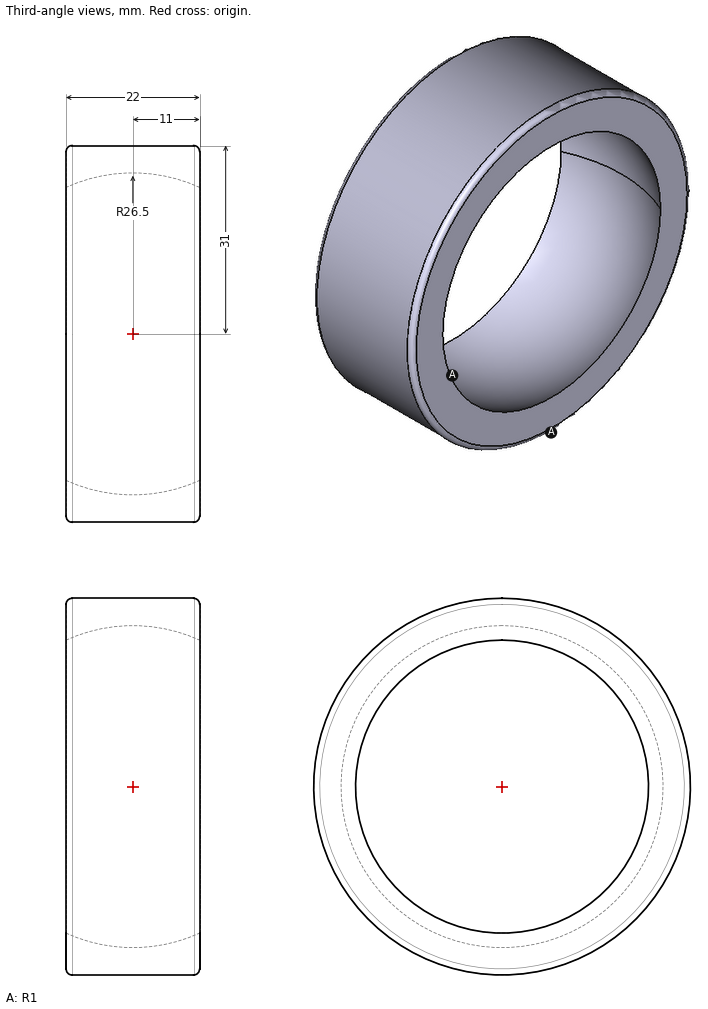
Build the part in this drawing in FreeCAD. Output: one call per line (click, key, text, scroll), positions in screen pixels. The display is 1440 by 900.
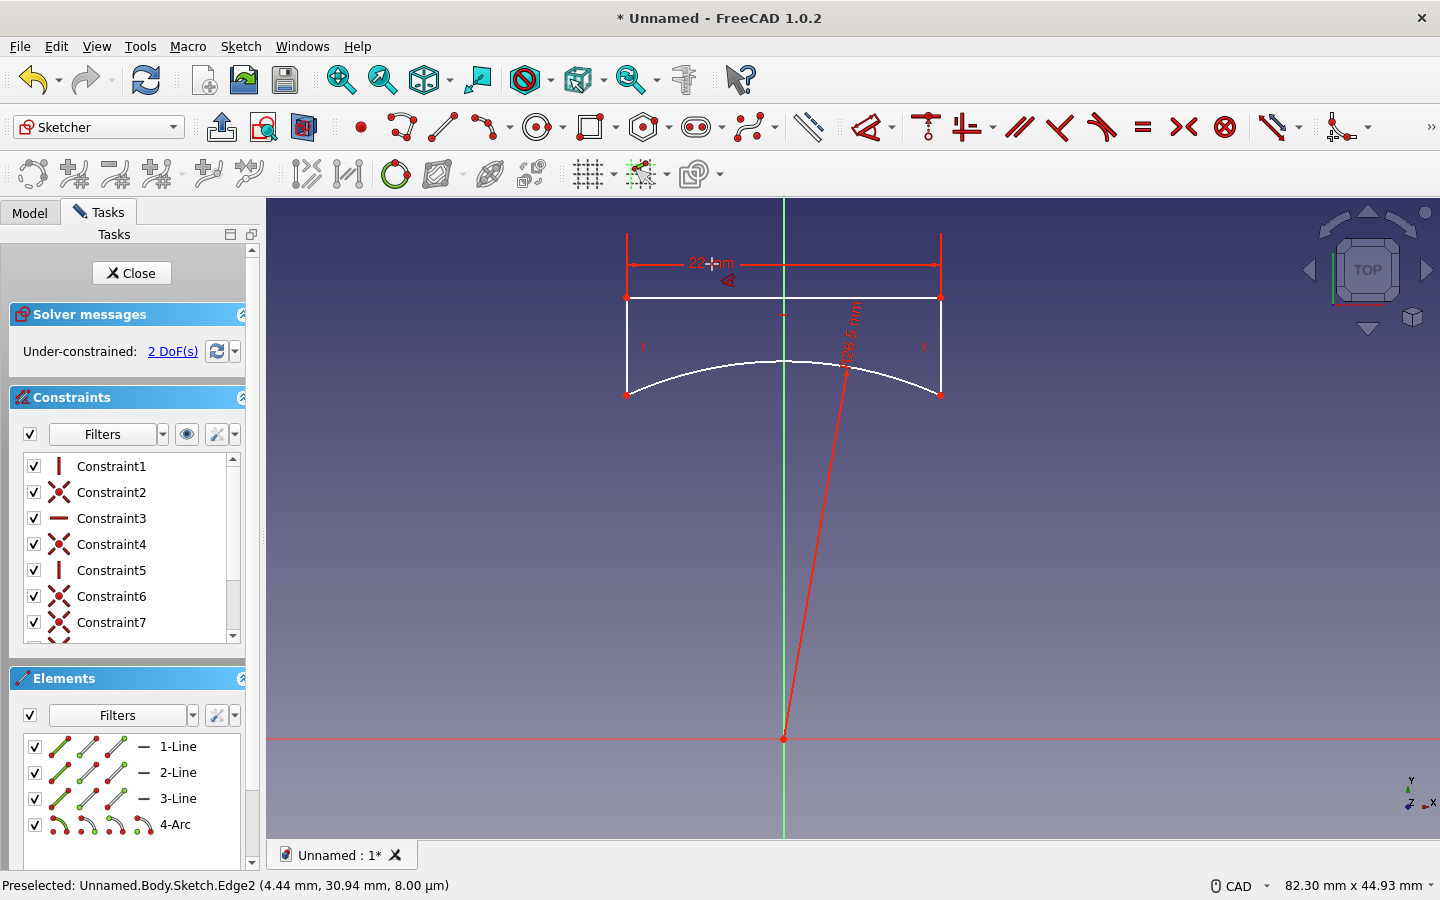
click(941, 396)
click(862, 773)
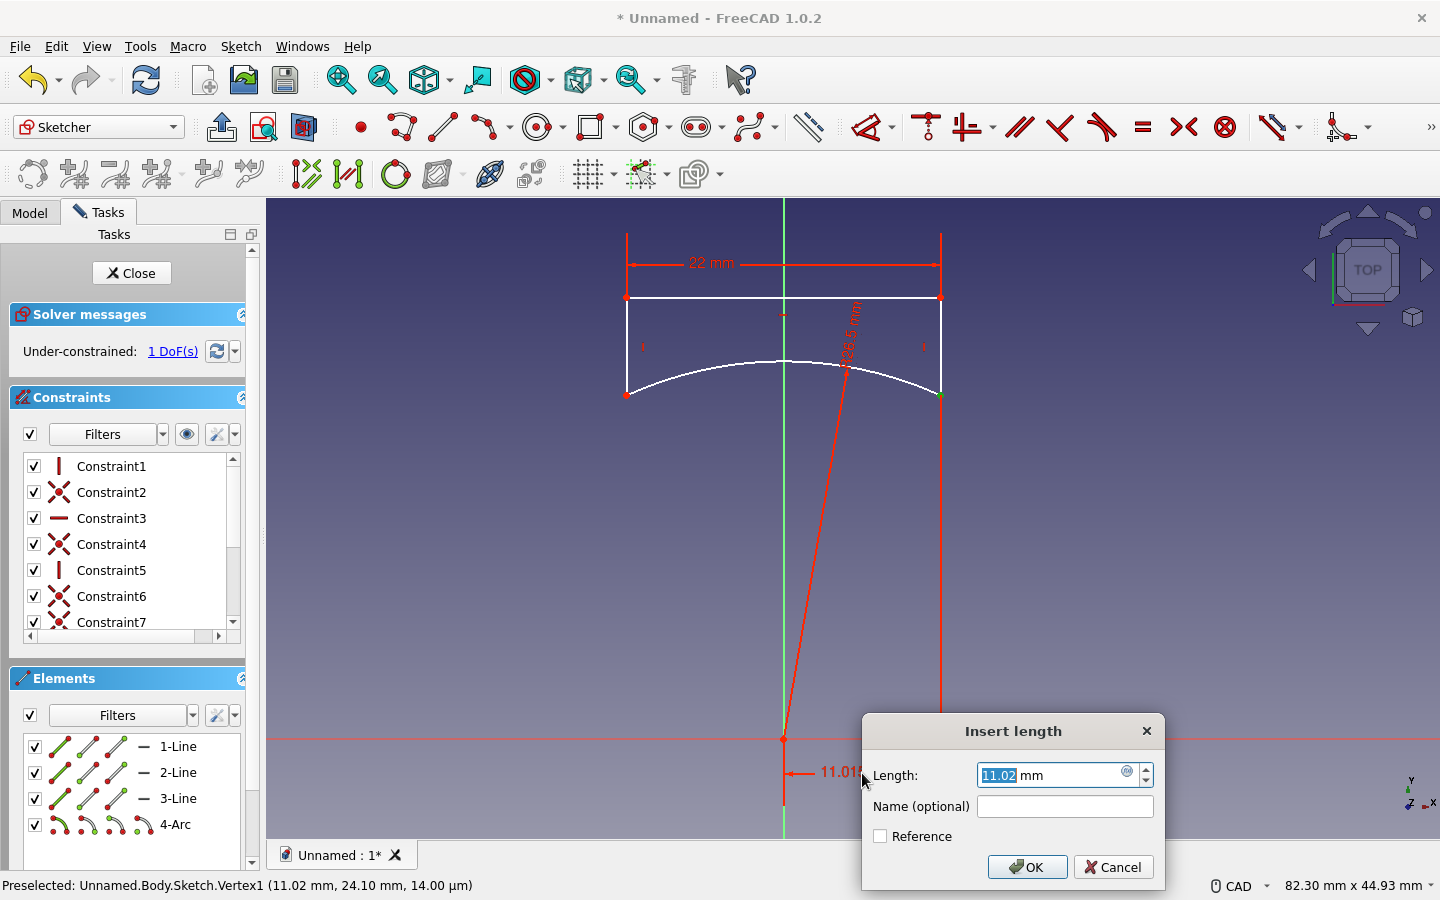
text(11)
key(Return)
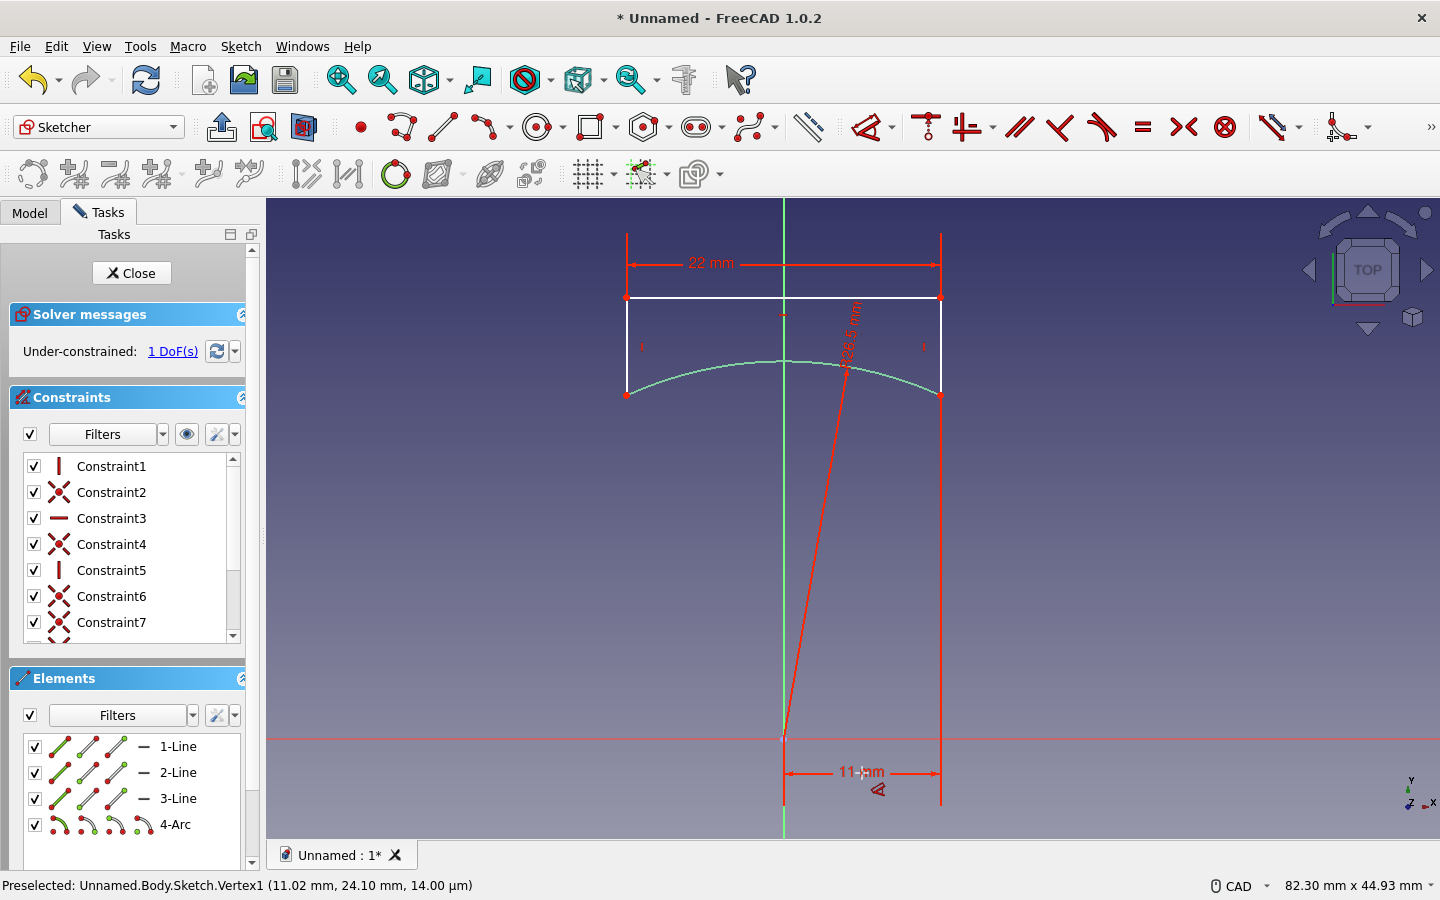
click(941, 298)
click(975, 519)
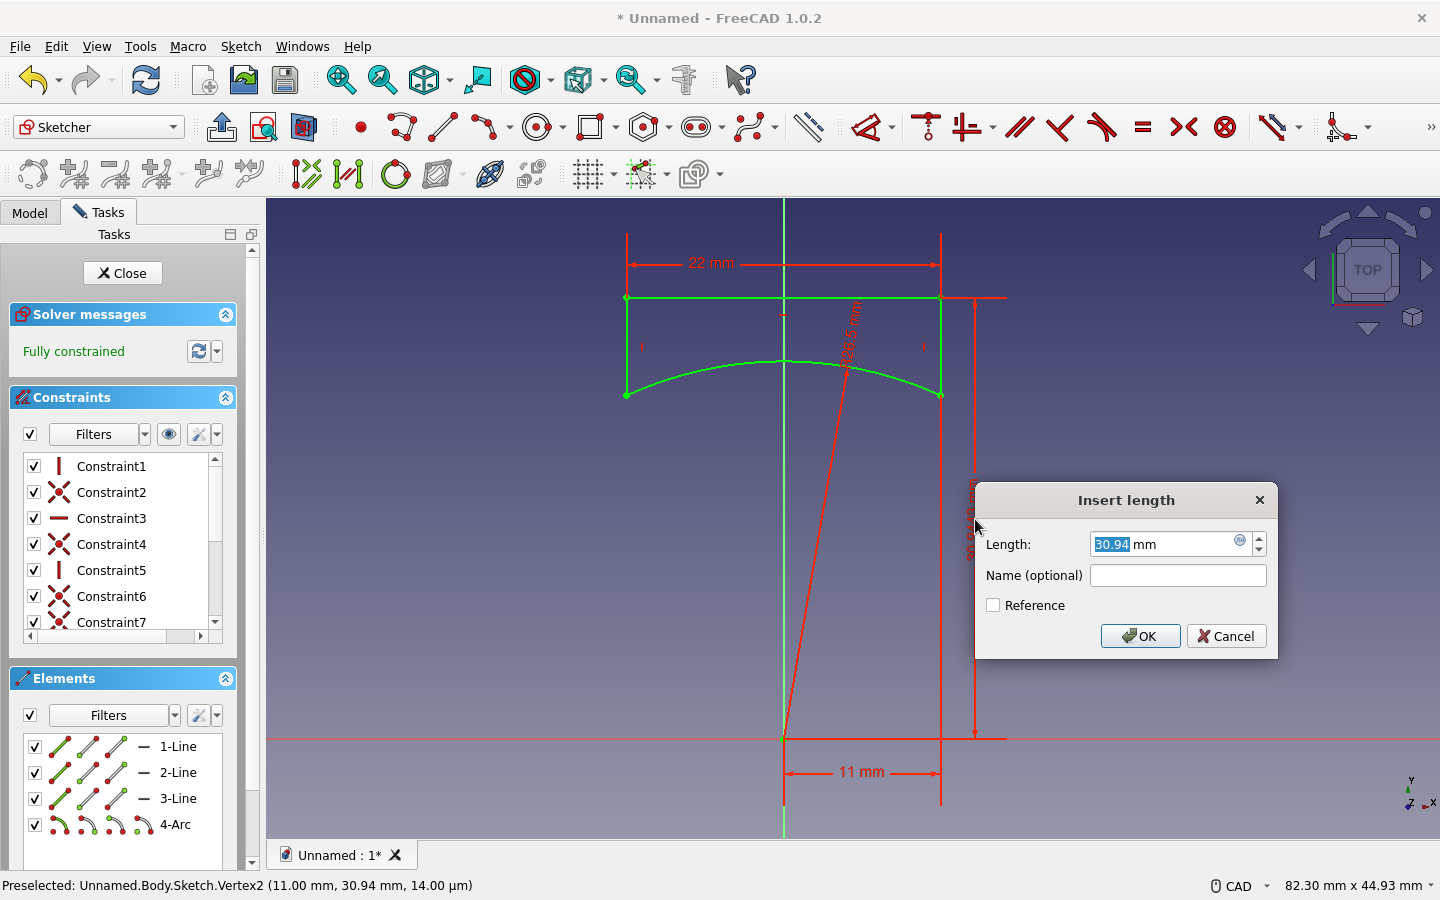
text(31)
key(Return)
key(Escape)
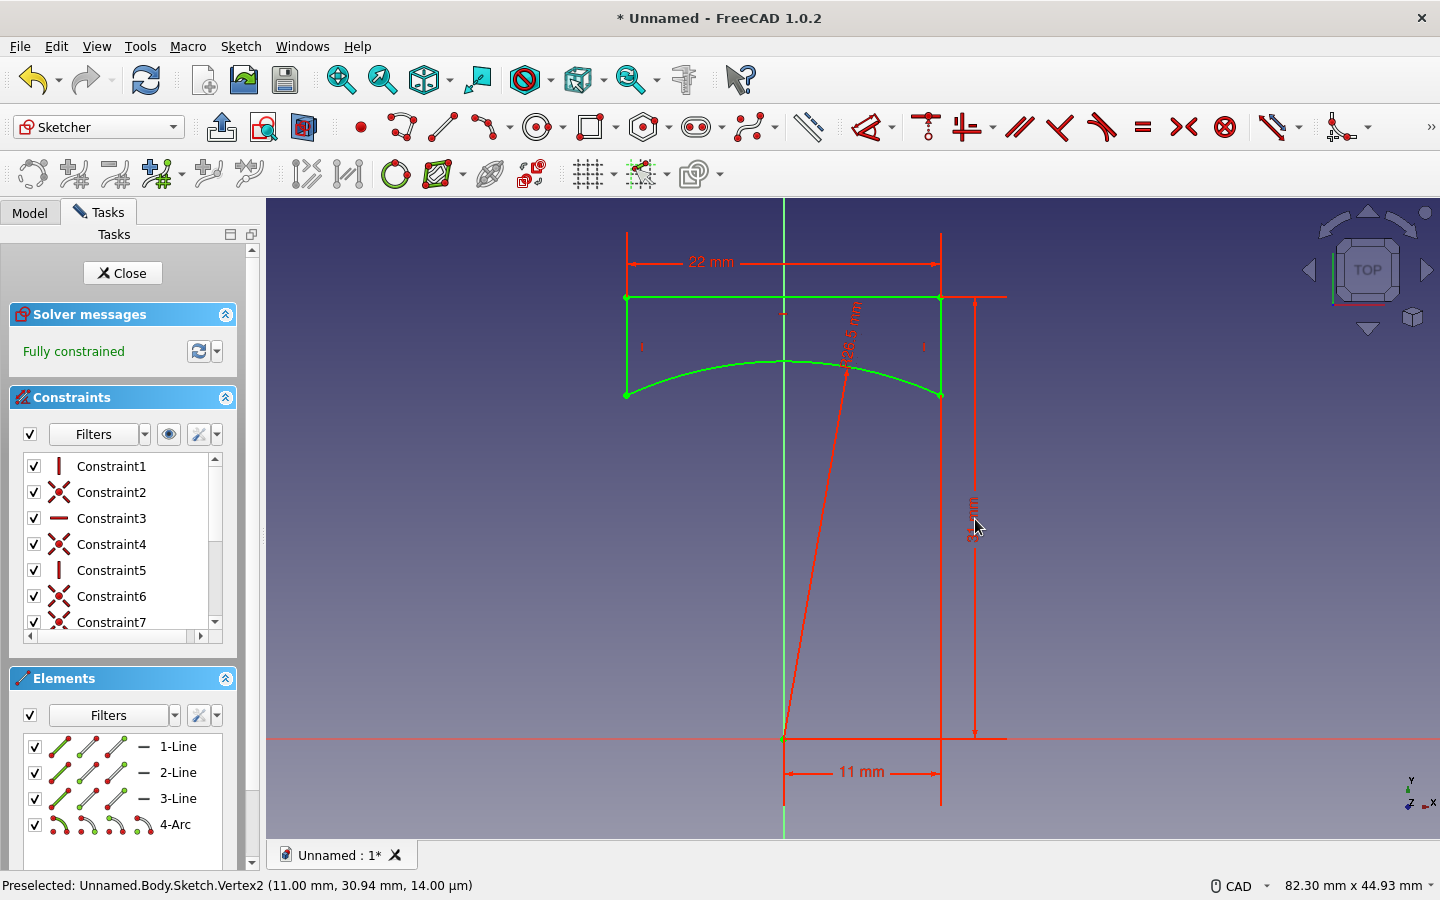
click(123, 273)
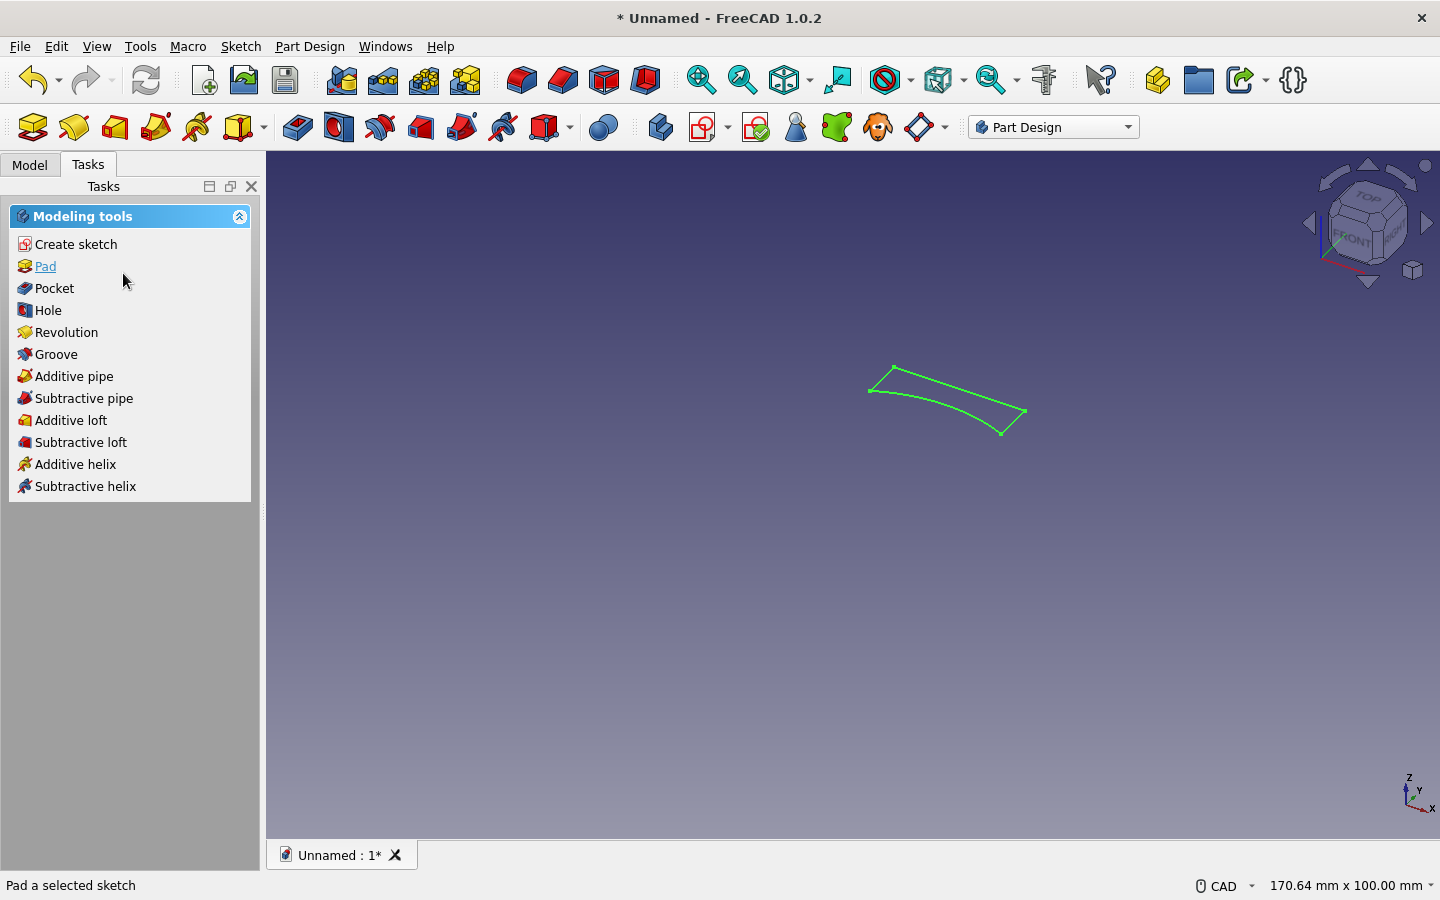
click(74, 128)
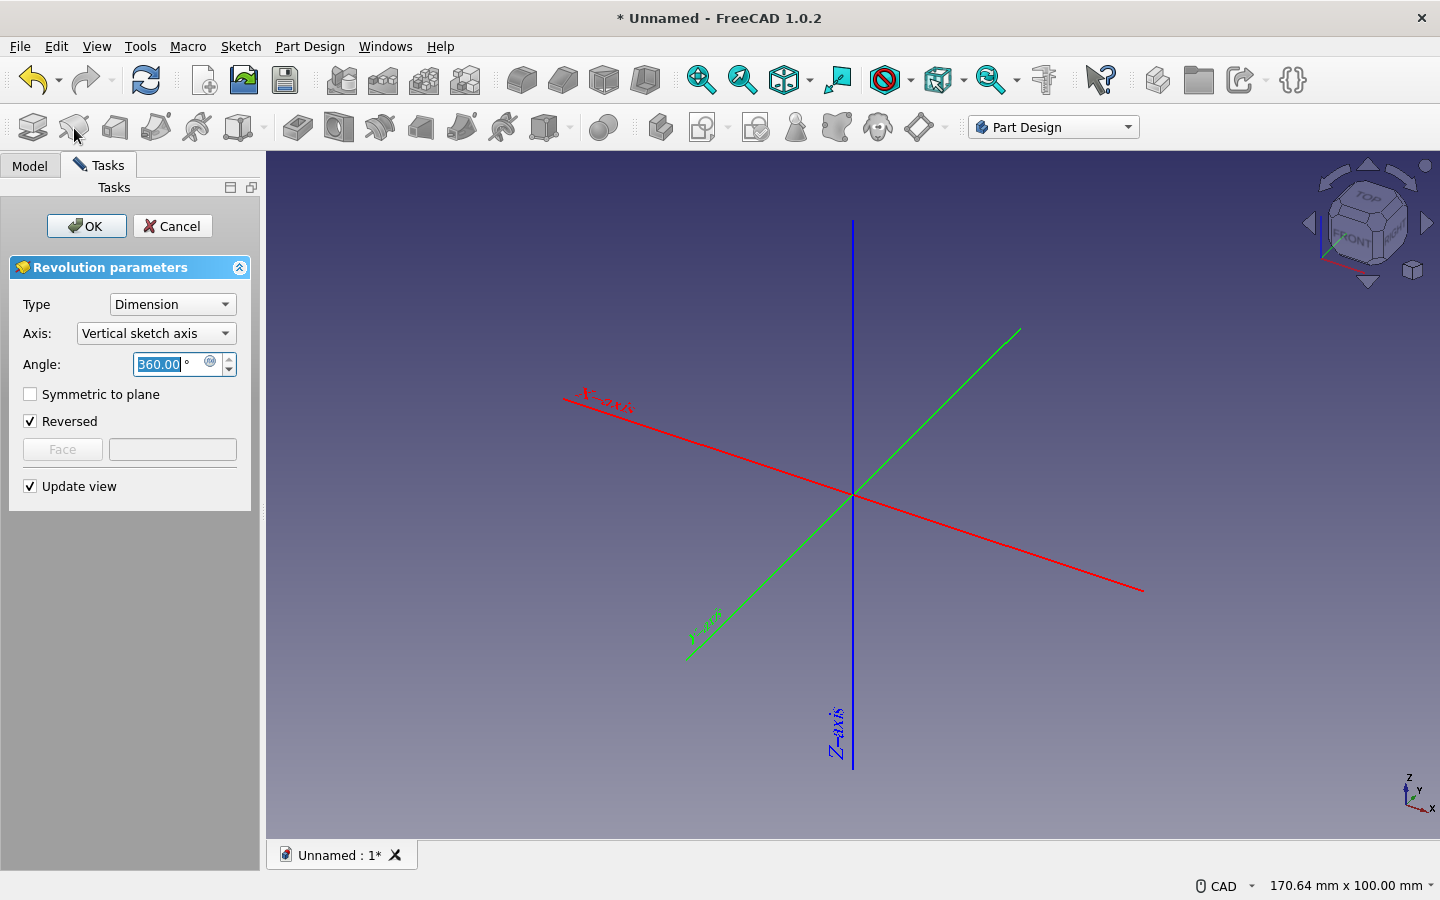
click(157, 334)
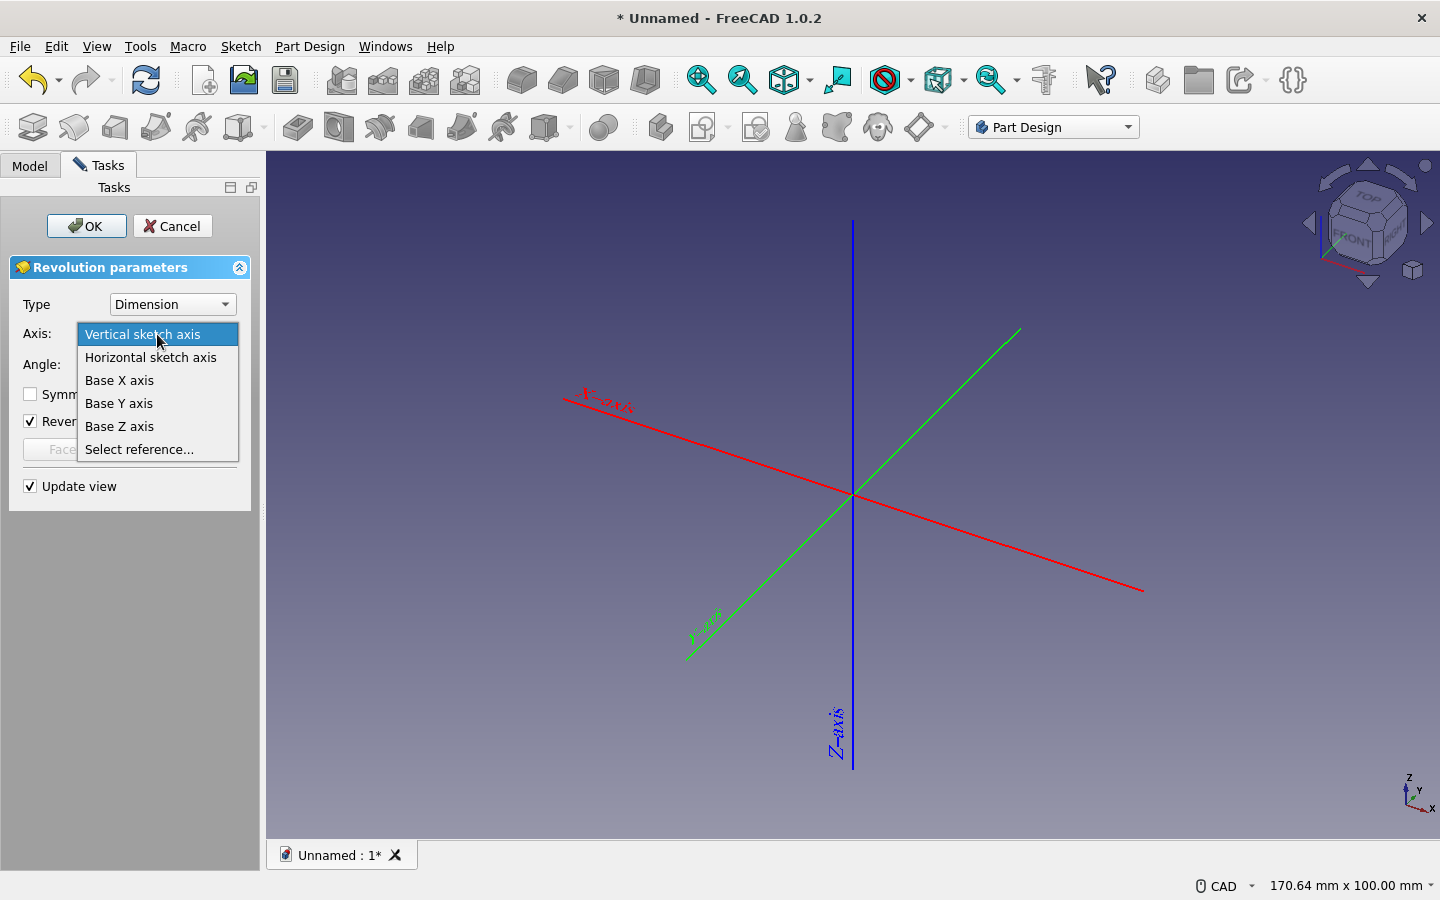
click(156, 358)